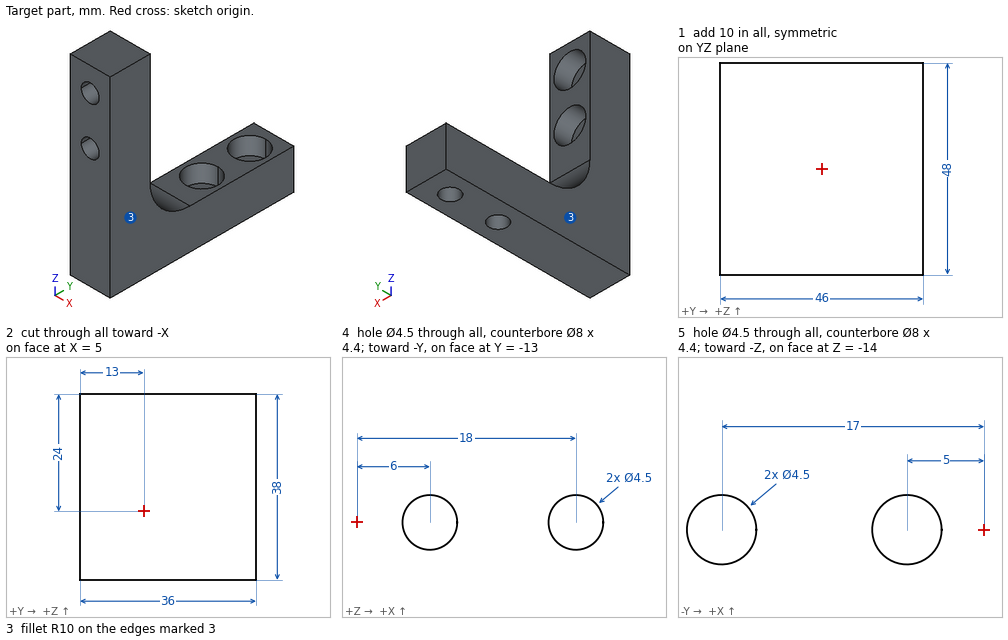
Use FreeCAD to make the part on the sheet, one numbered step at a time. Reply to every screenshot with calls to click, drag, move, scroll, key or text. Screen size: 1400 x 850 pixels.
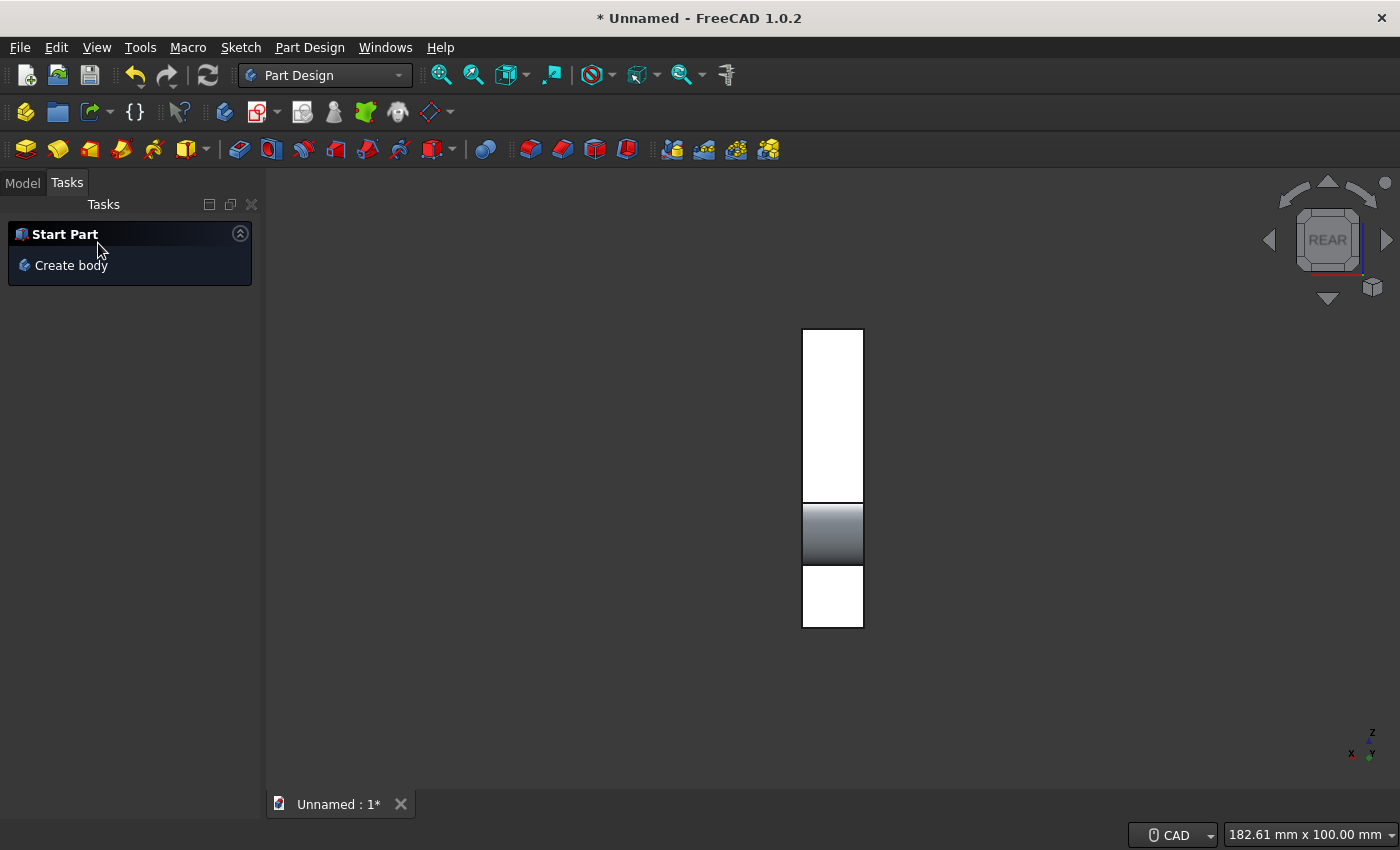
click(833, 465)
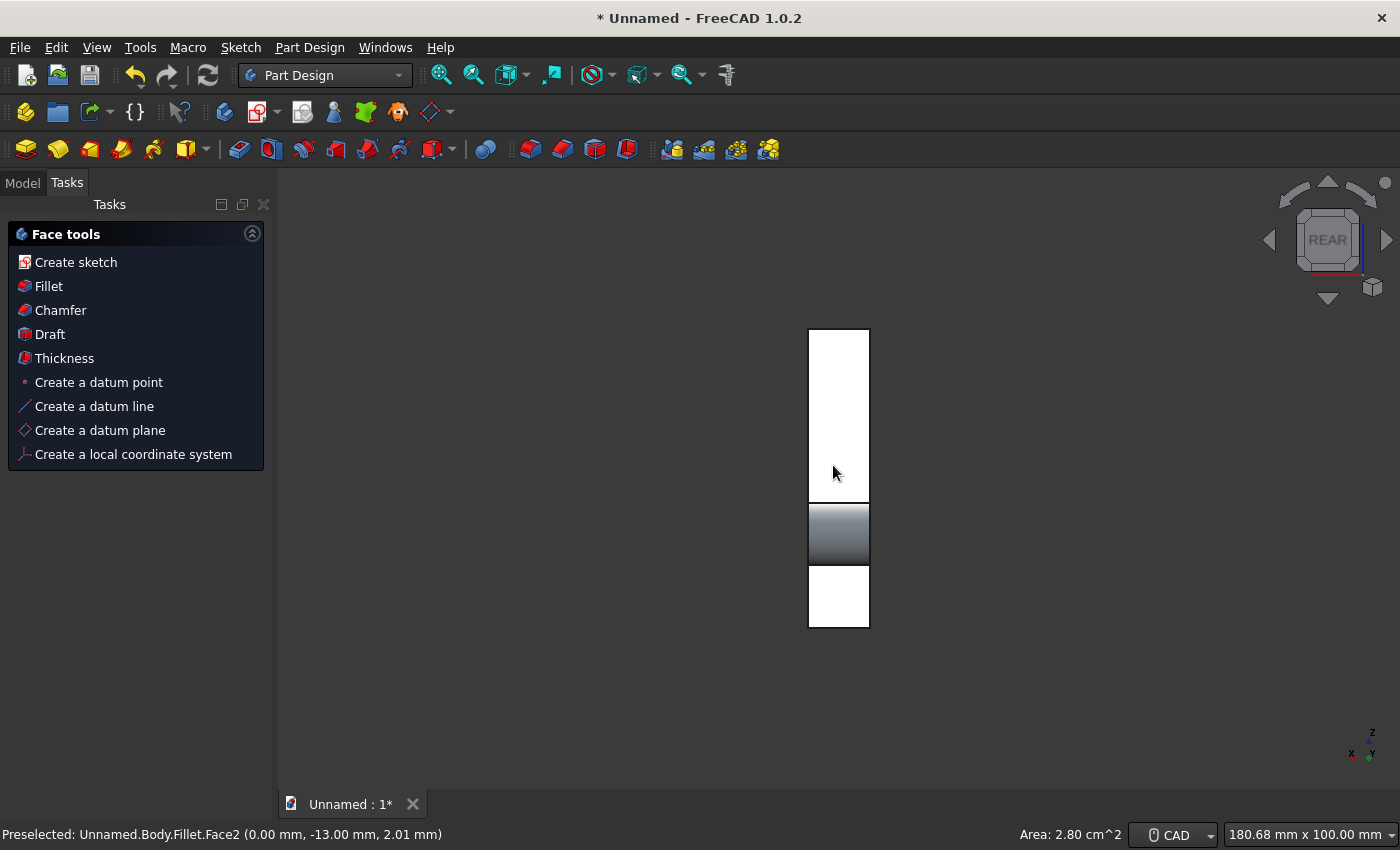
click(258, 112)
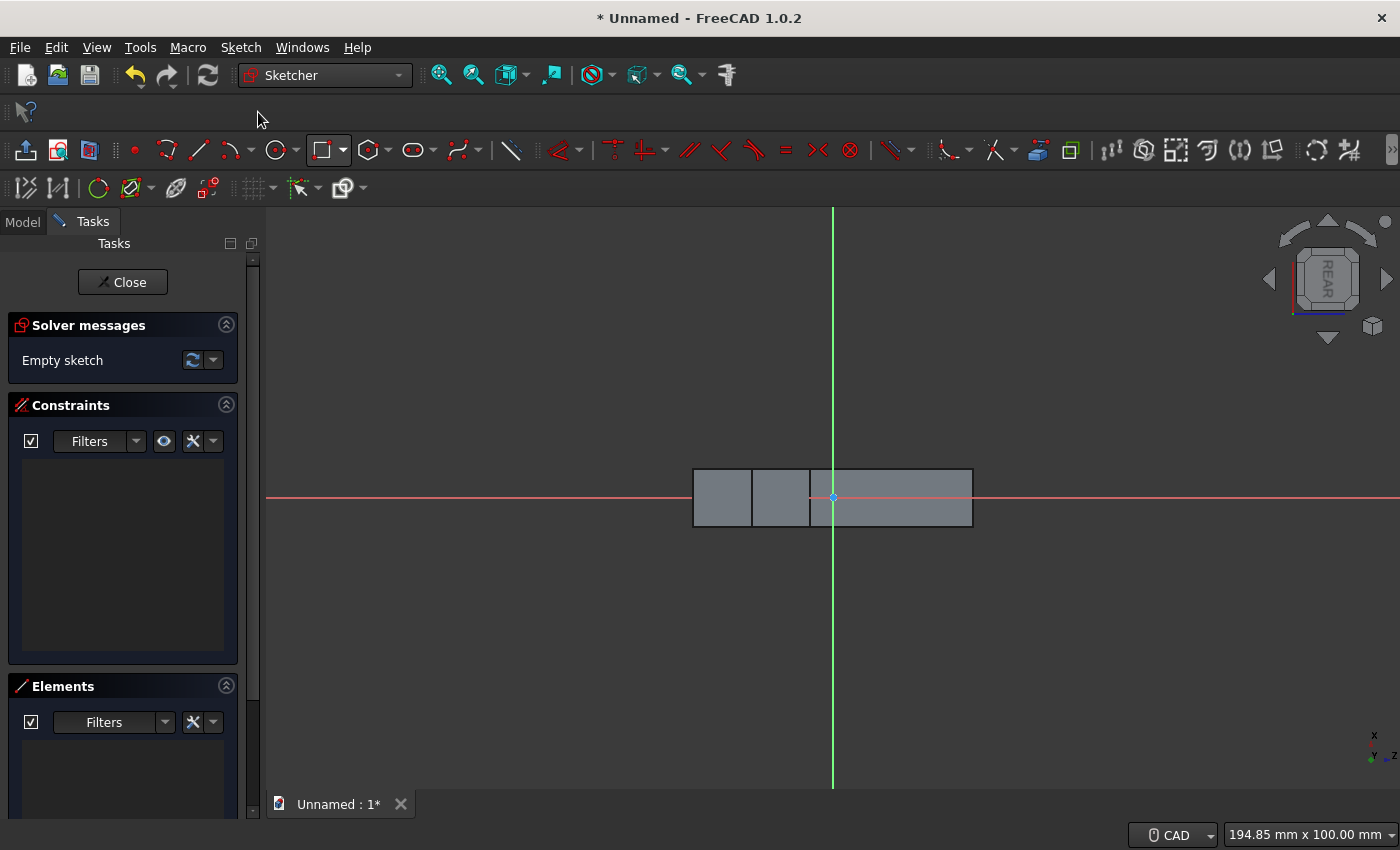
scroll(917, 498, up, 9)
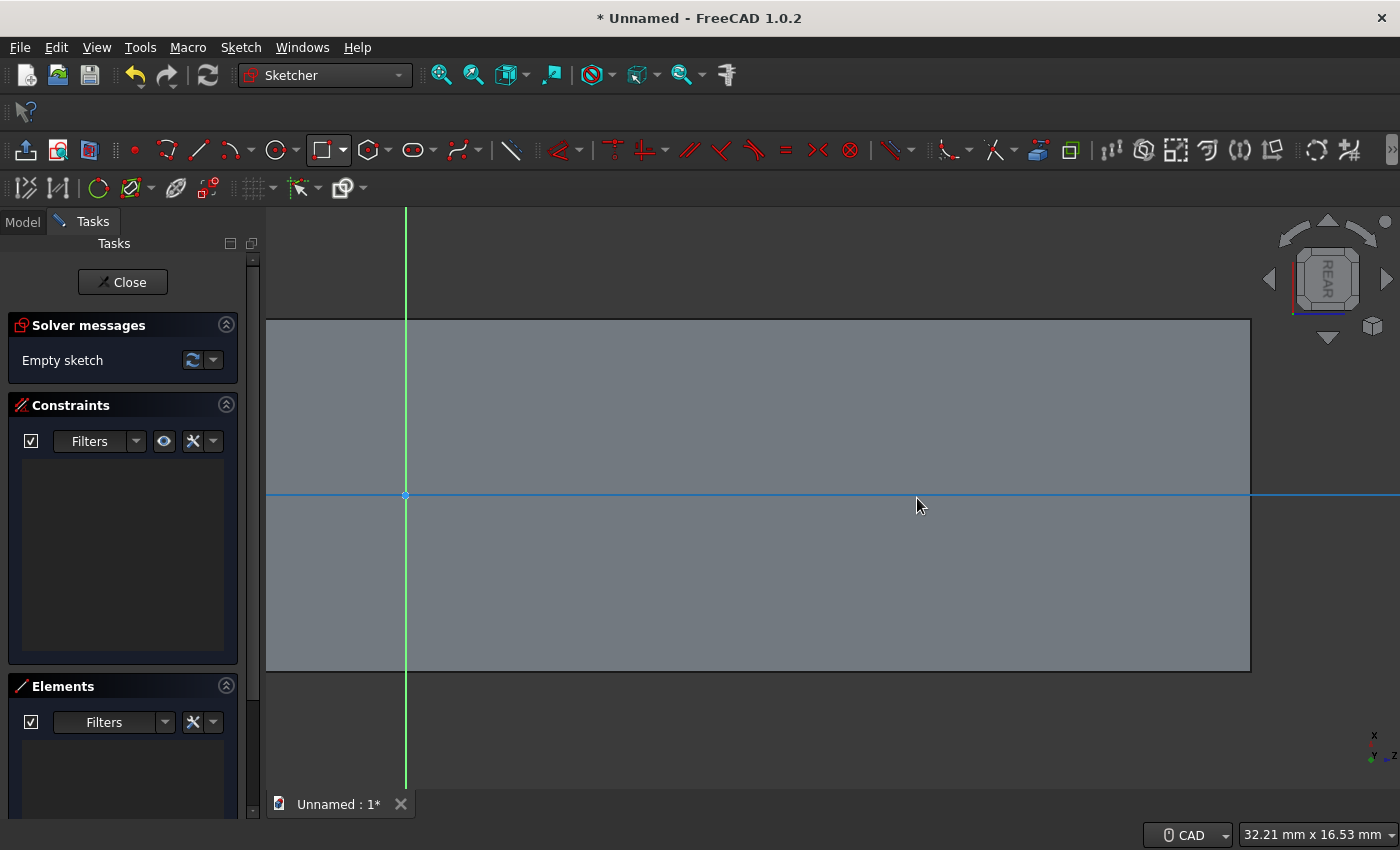
click(276, 150)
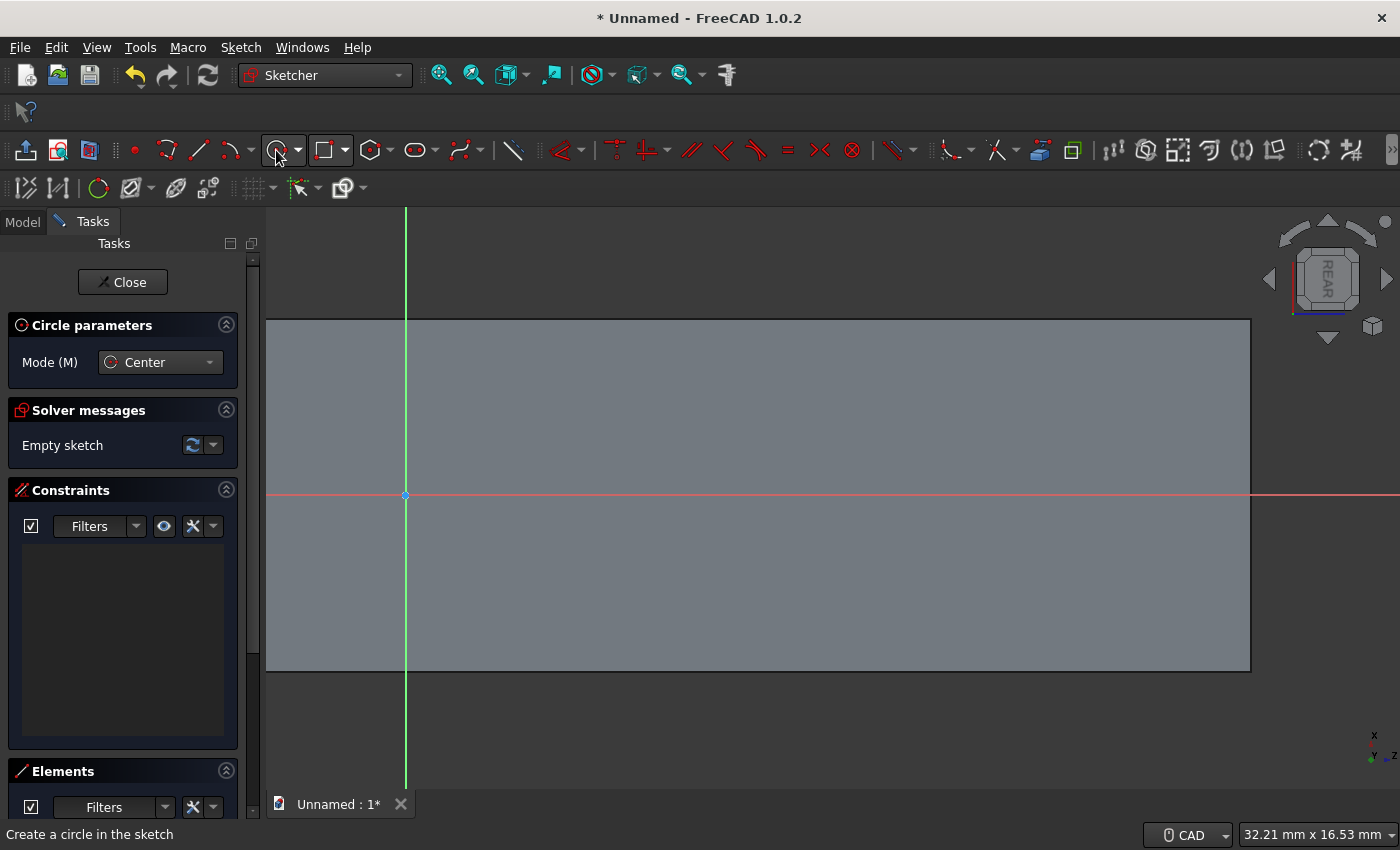
click(1040, 495)
move(1096, 439)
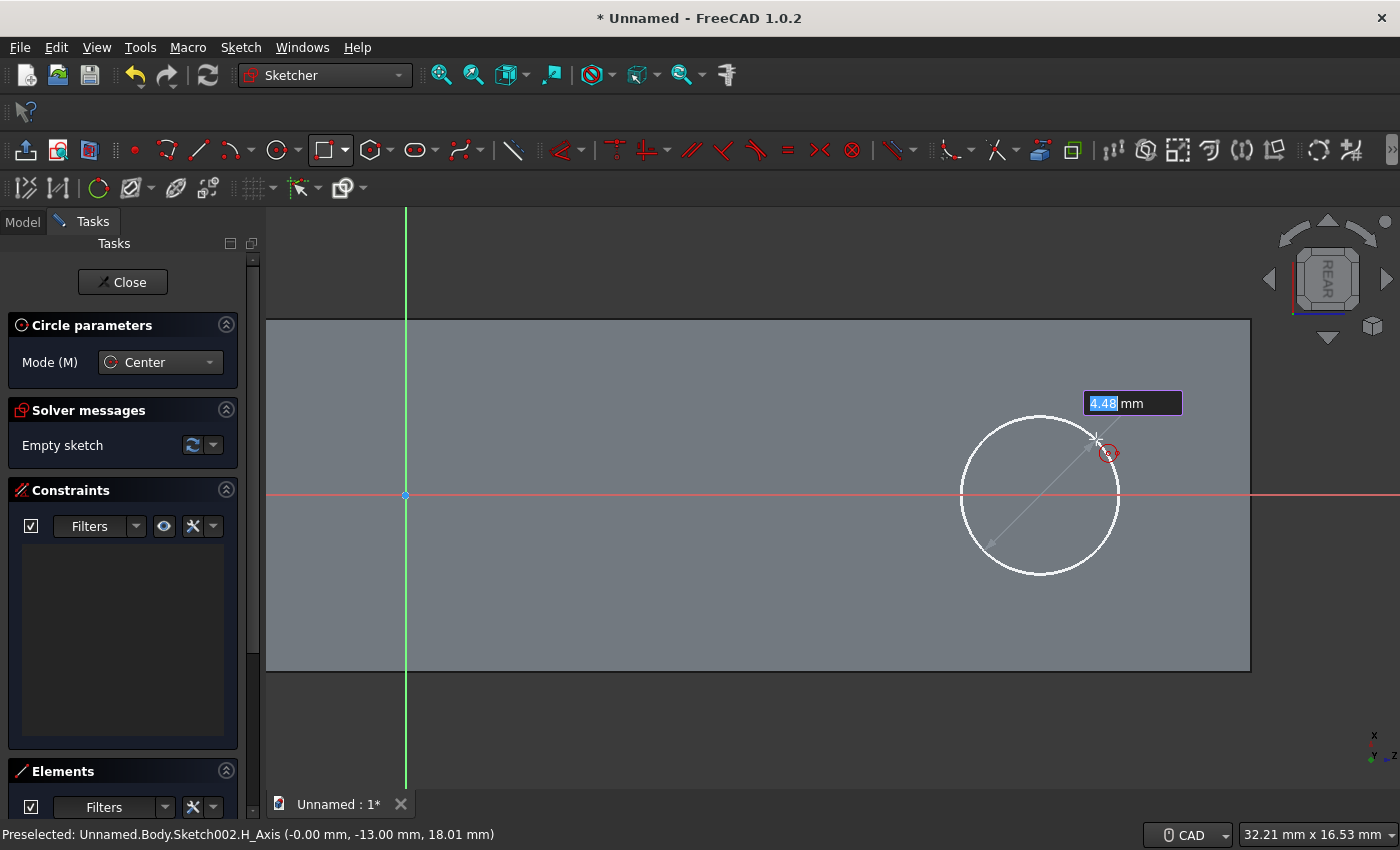
text(4.5)
key(Return)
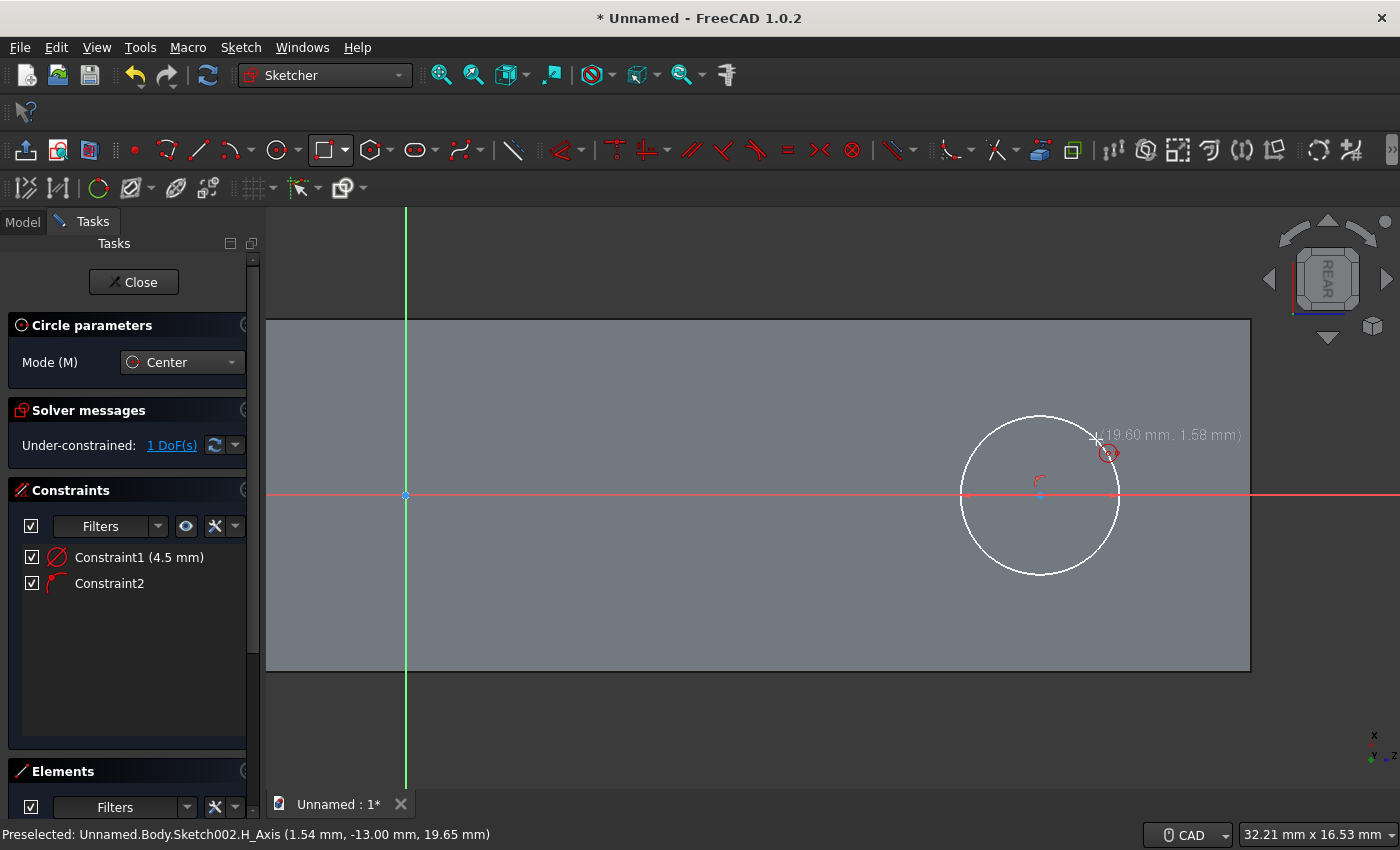
click(617, 495)
move(673, 439)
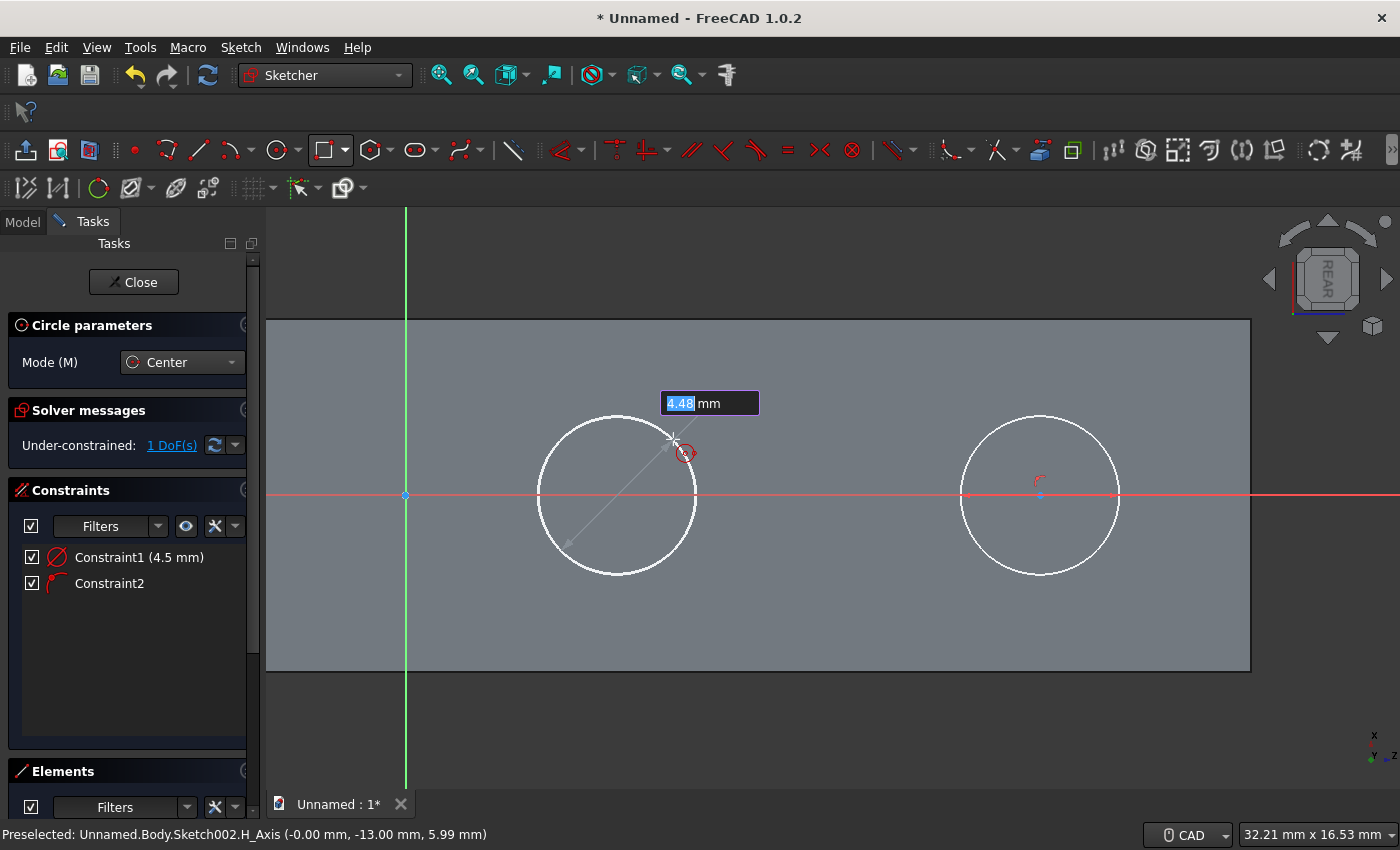
text(4.5)
key(Return)
key(Escape)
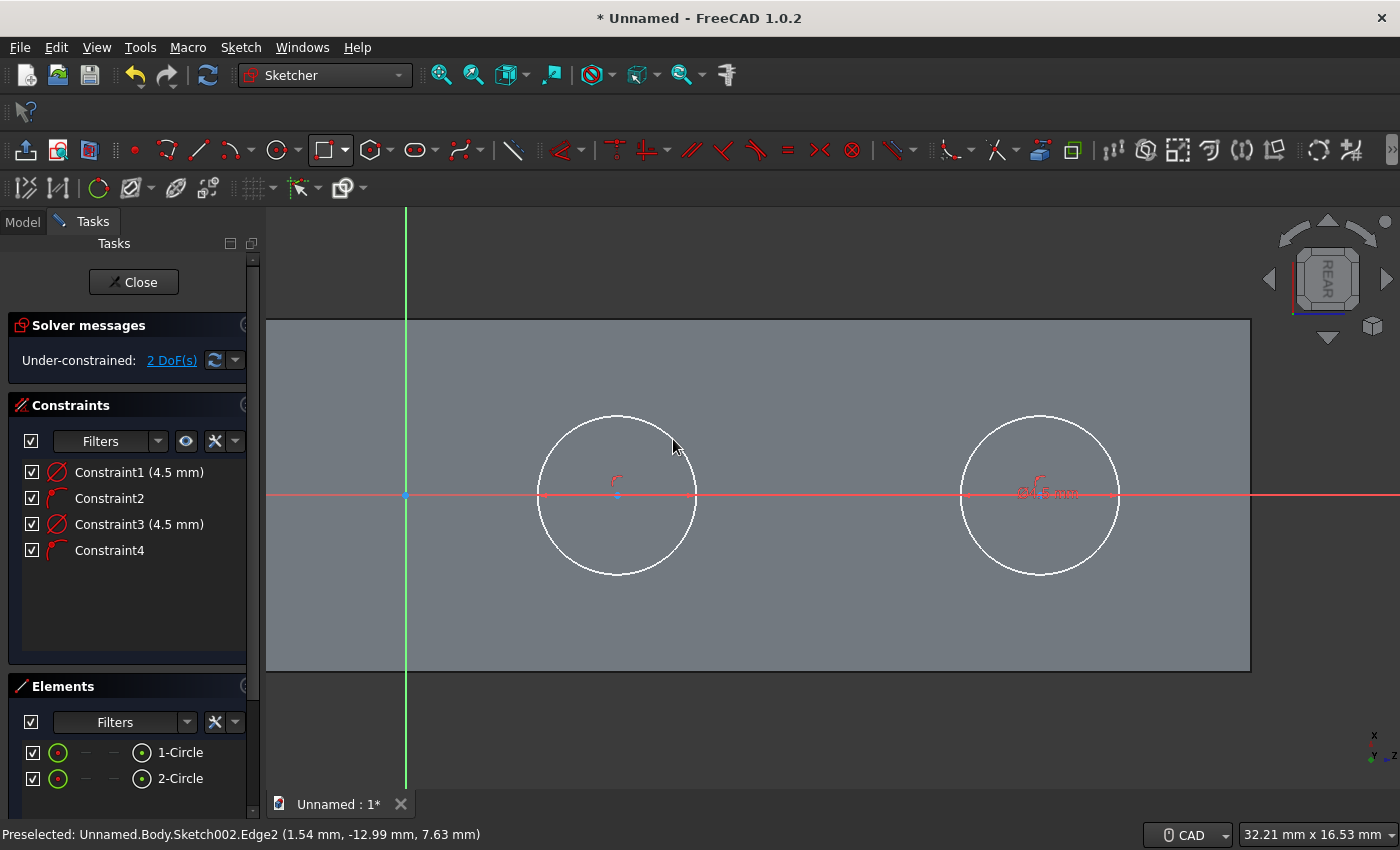
click(560, 150)